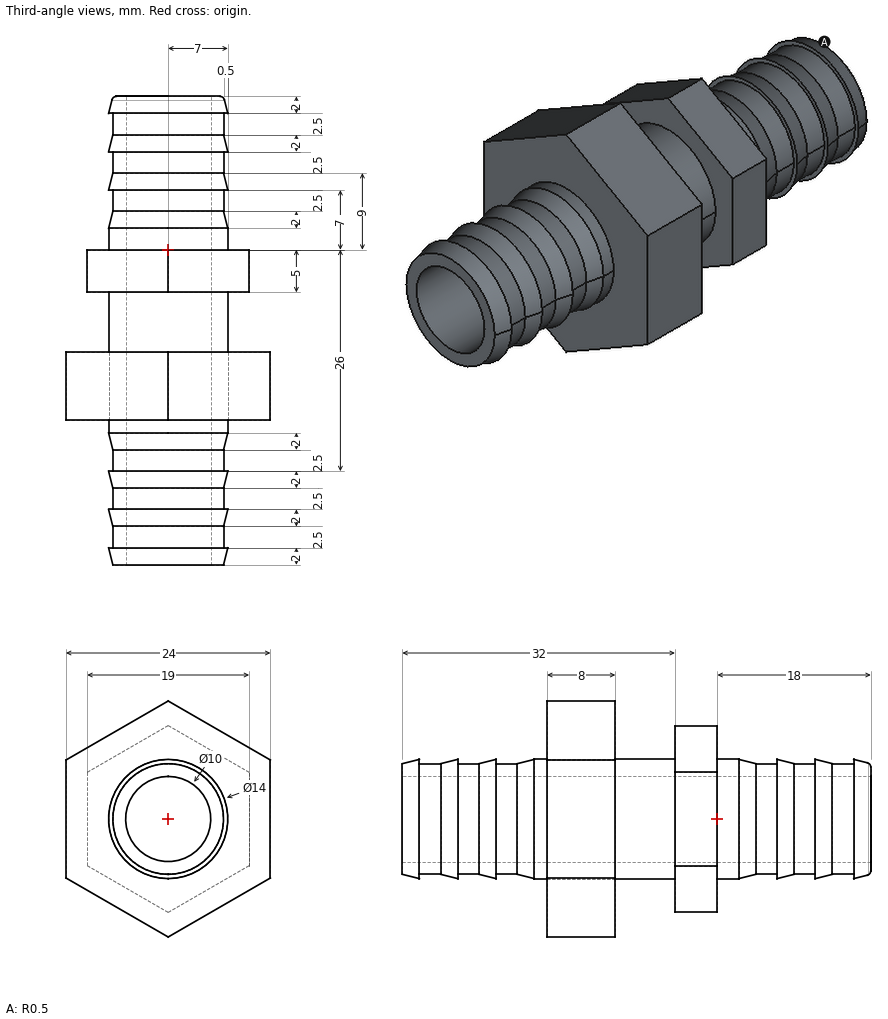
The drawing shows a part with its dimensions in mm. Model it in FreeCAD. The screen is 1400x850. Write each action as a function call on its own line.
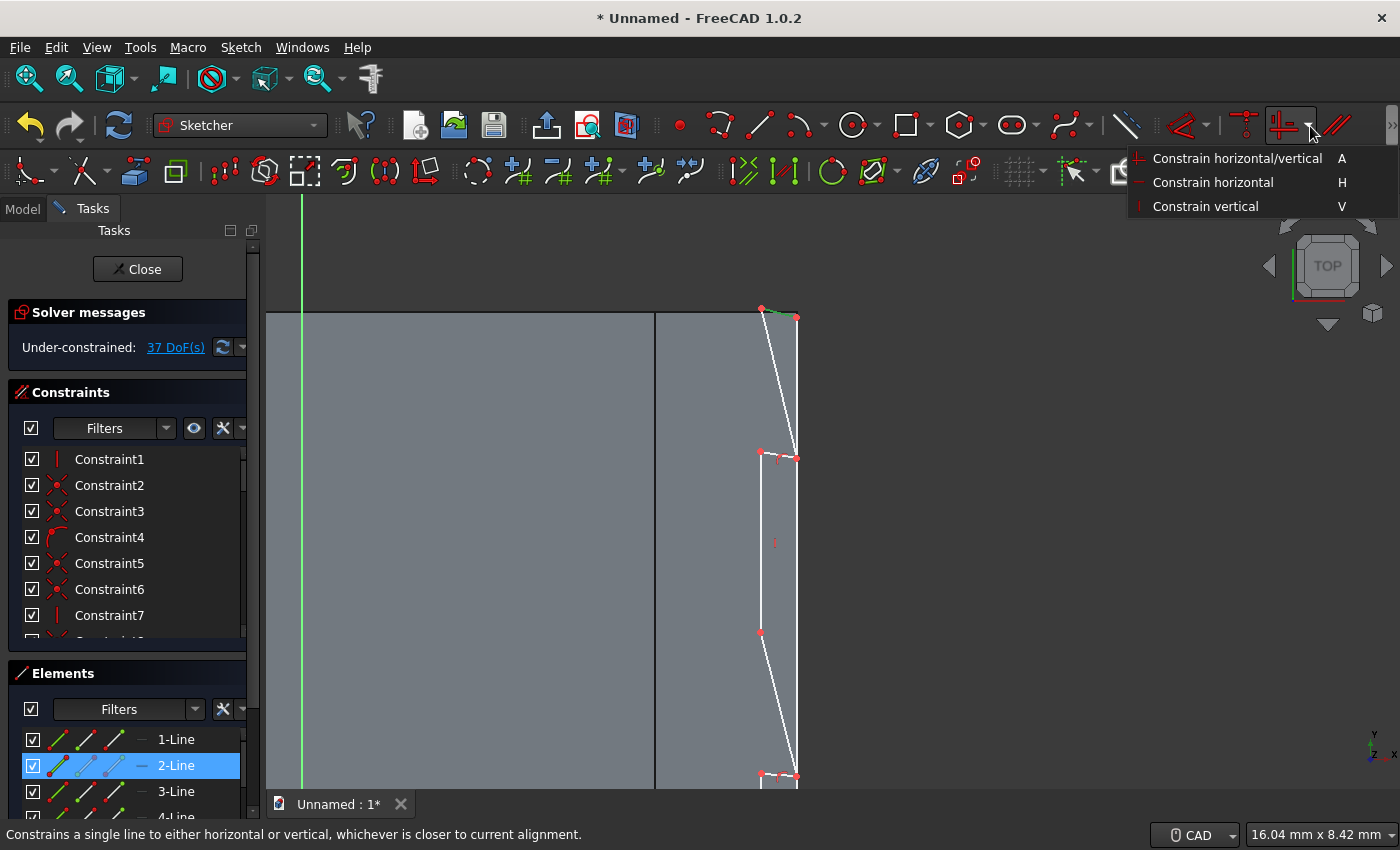
click(1263, 182)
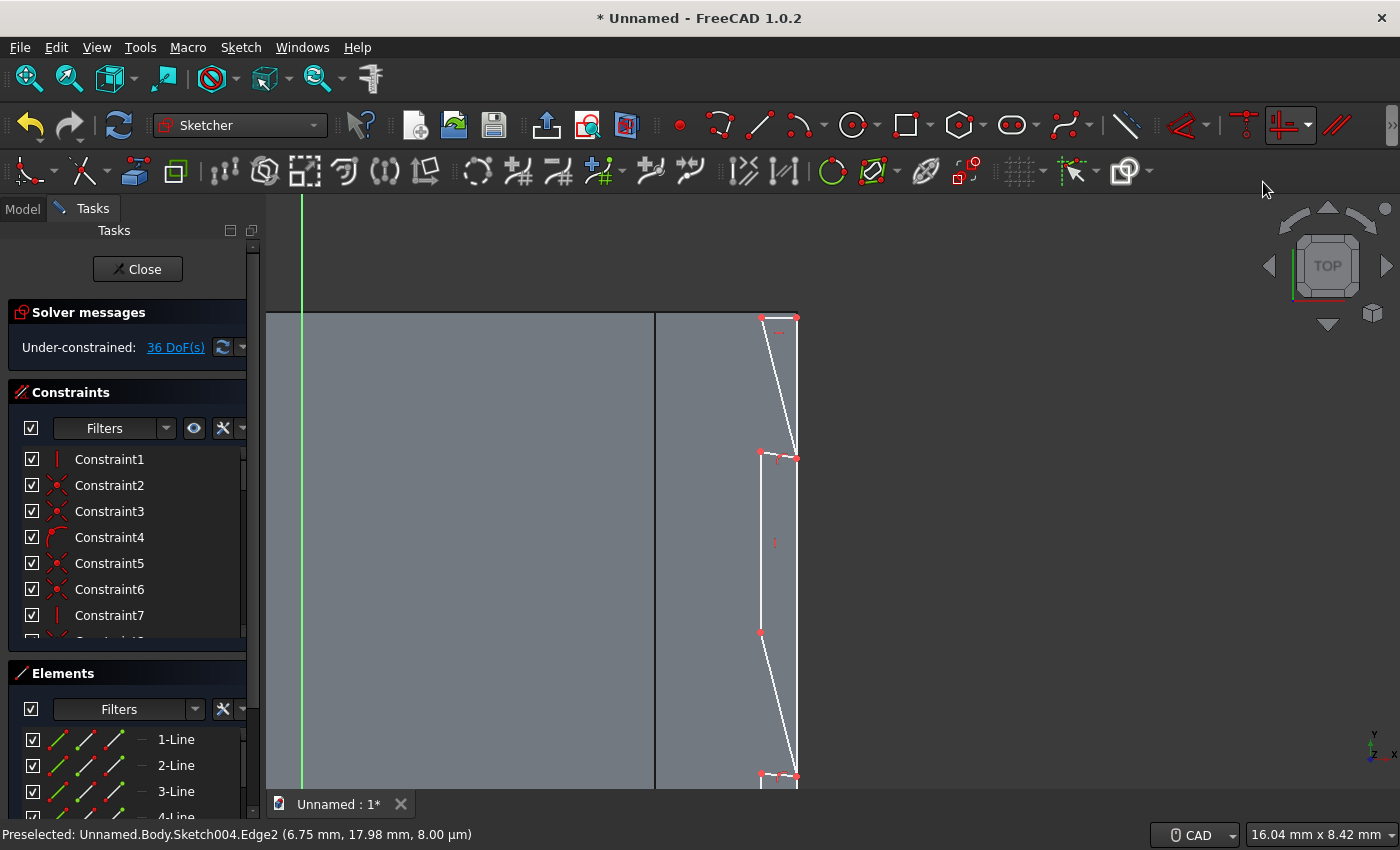
scroll(786, 456, up, 2)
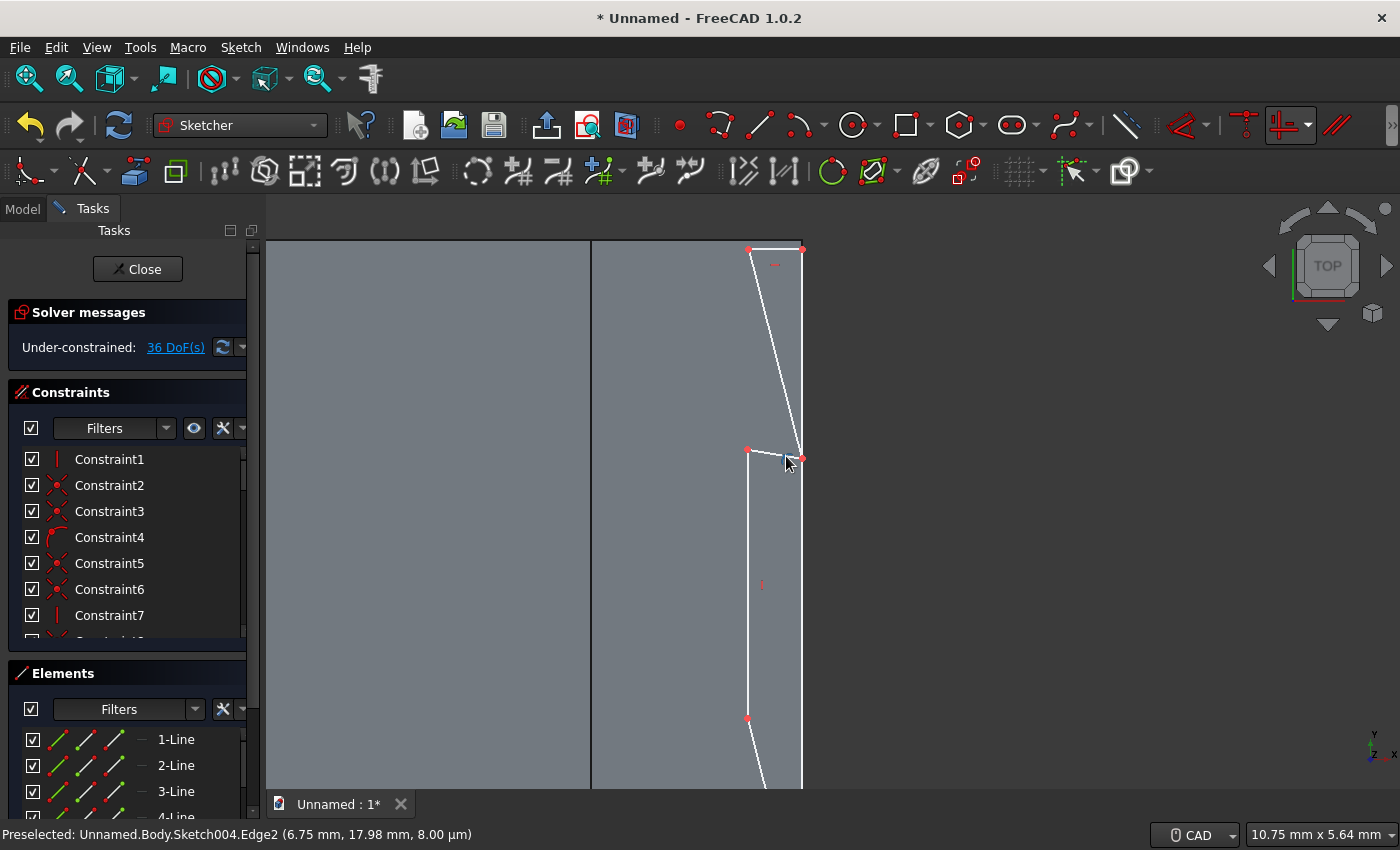
click(764, 452)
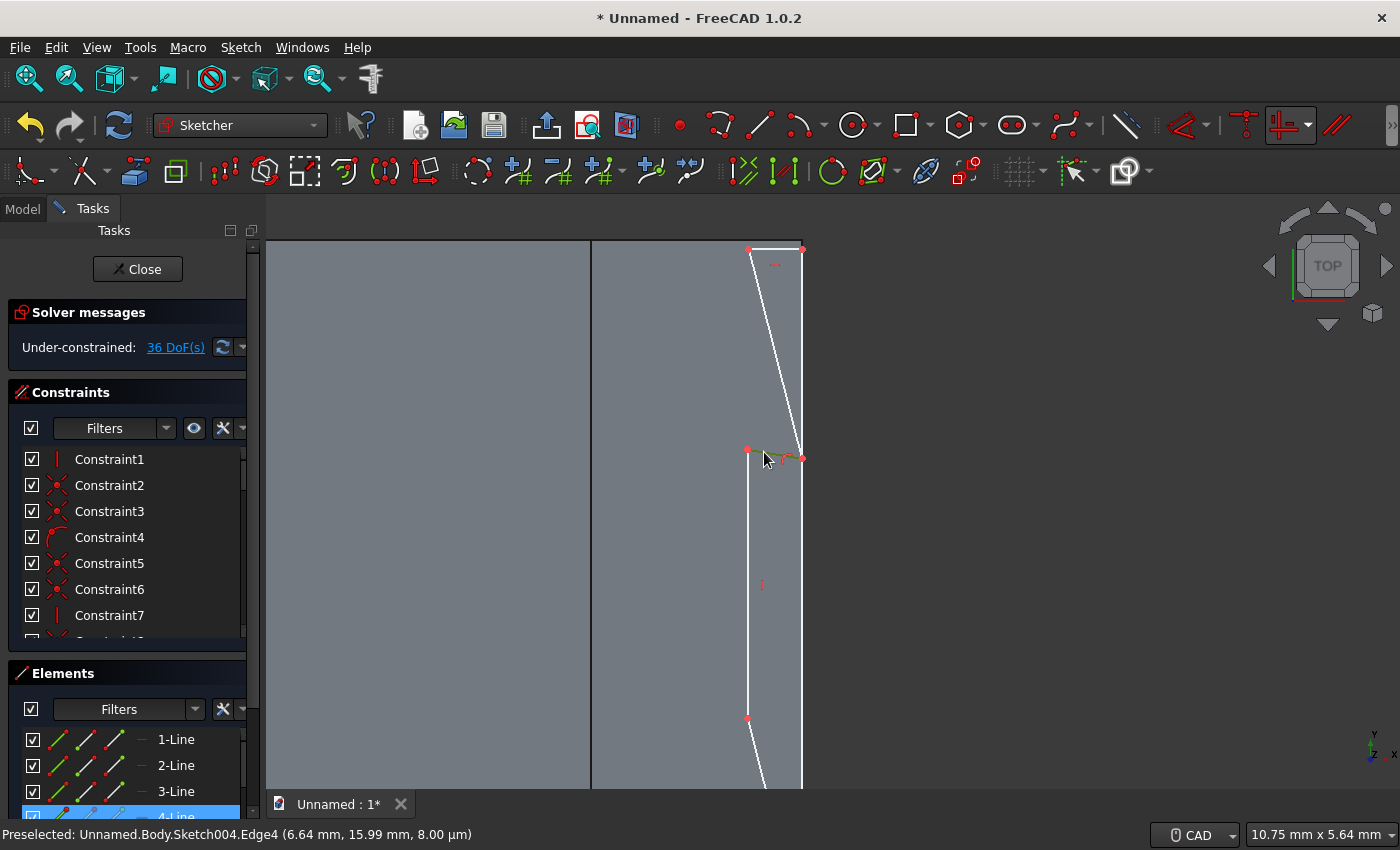
click(1310, 126)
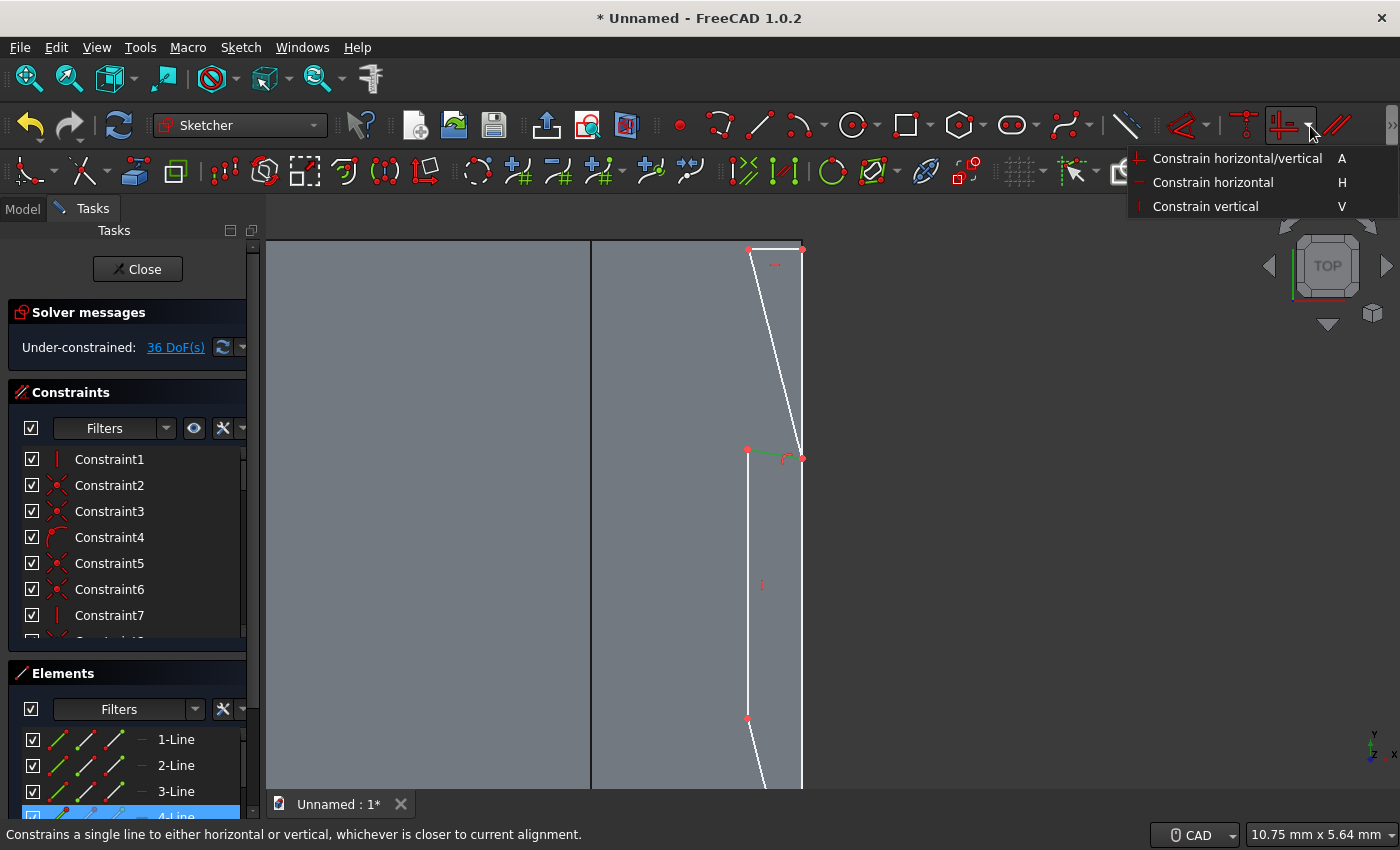
click(1263, 182)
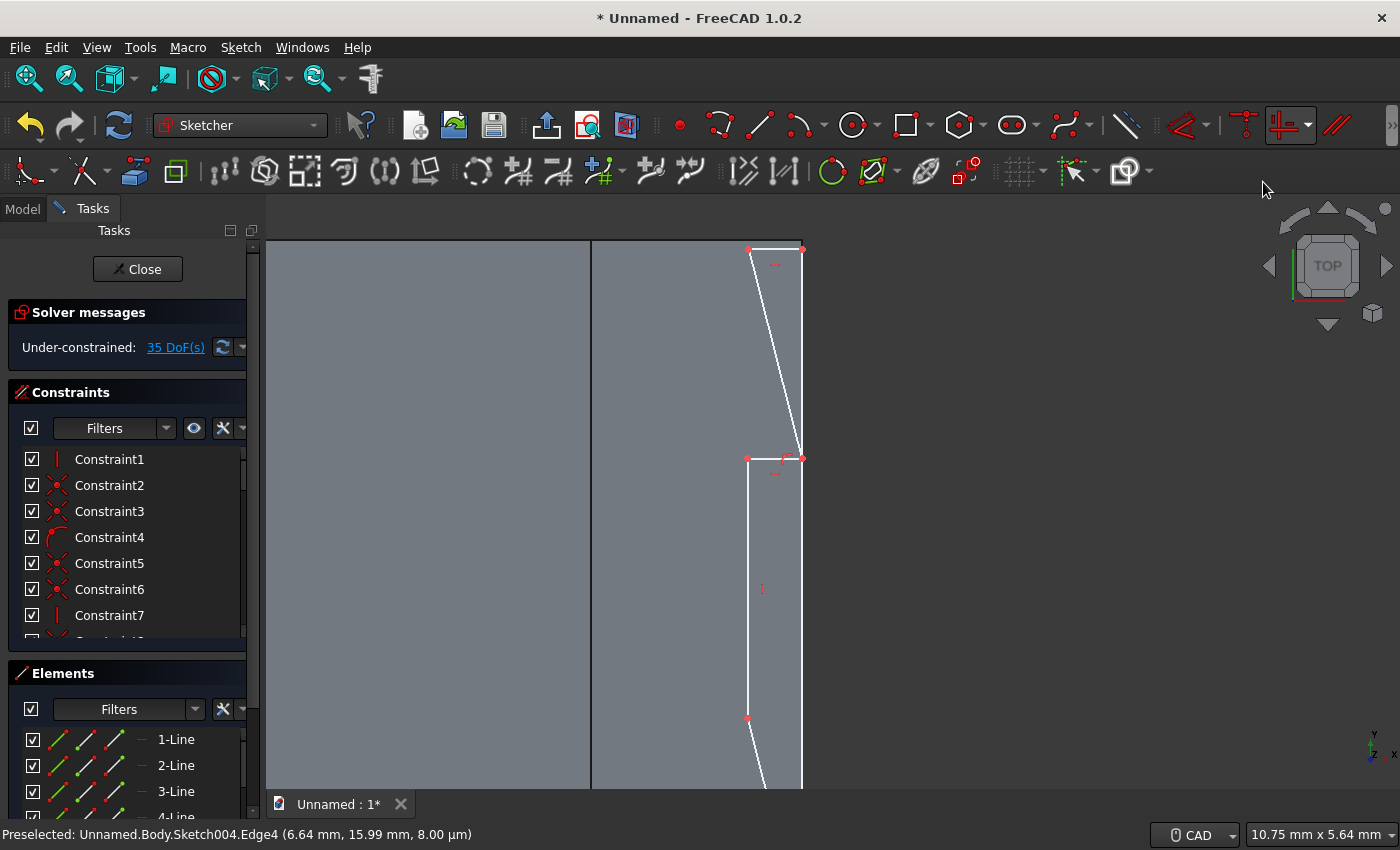
scroll(786, 320, down, 14)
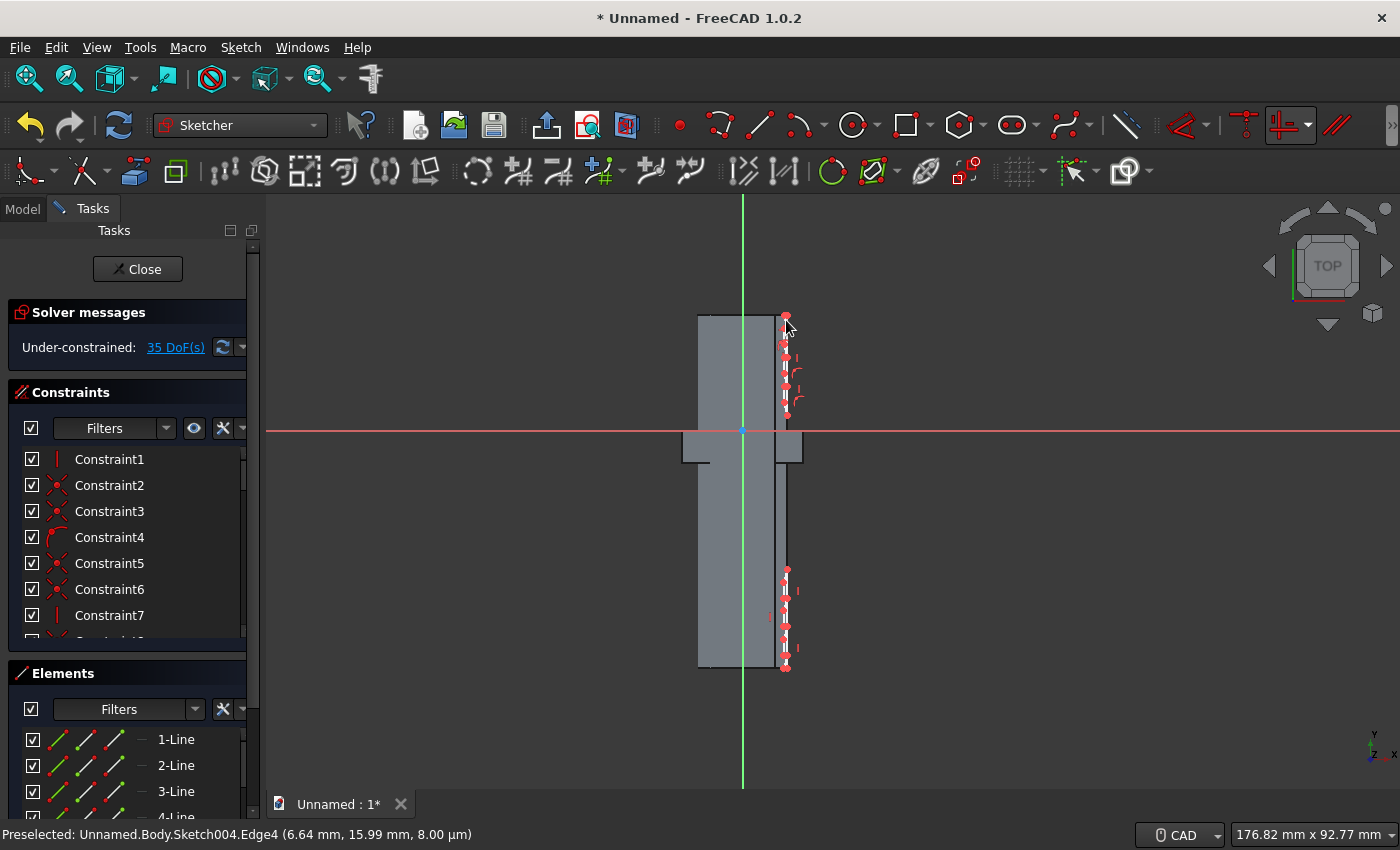
scroll(786, 357, up, 14)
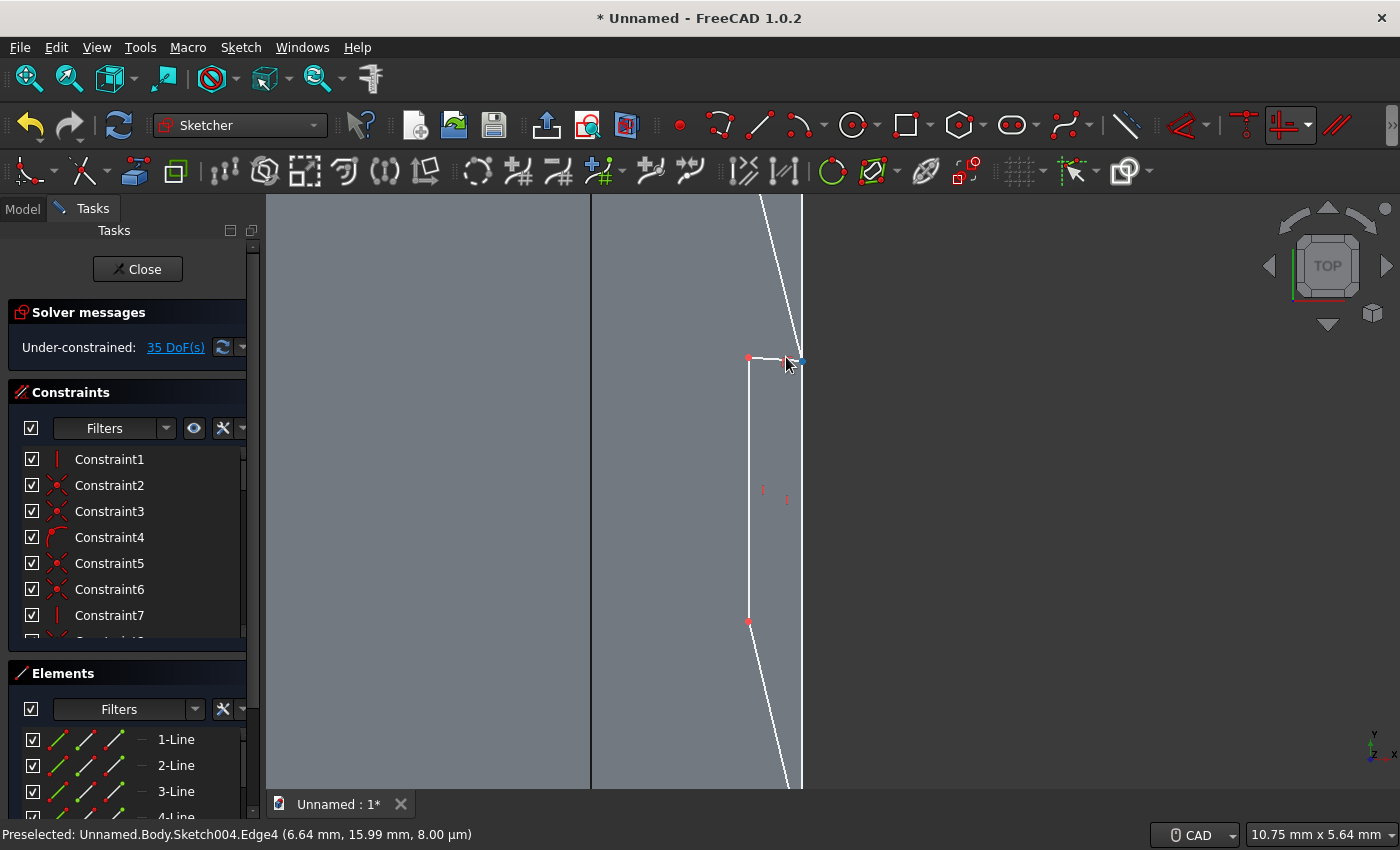
click(765, 359)